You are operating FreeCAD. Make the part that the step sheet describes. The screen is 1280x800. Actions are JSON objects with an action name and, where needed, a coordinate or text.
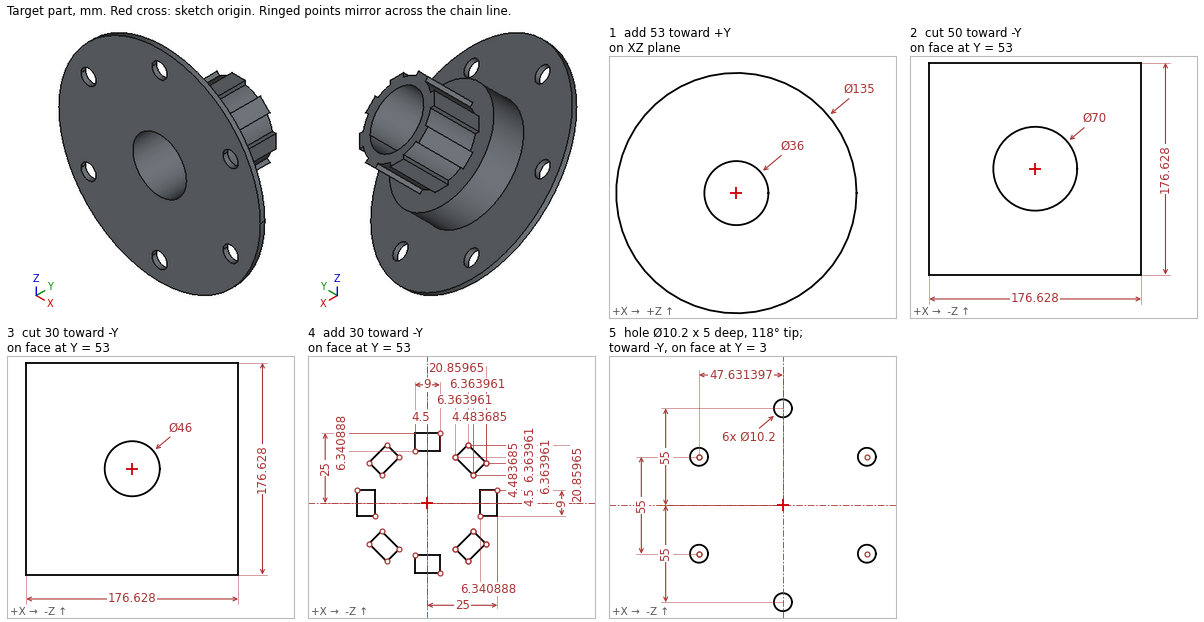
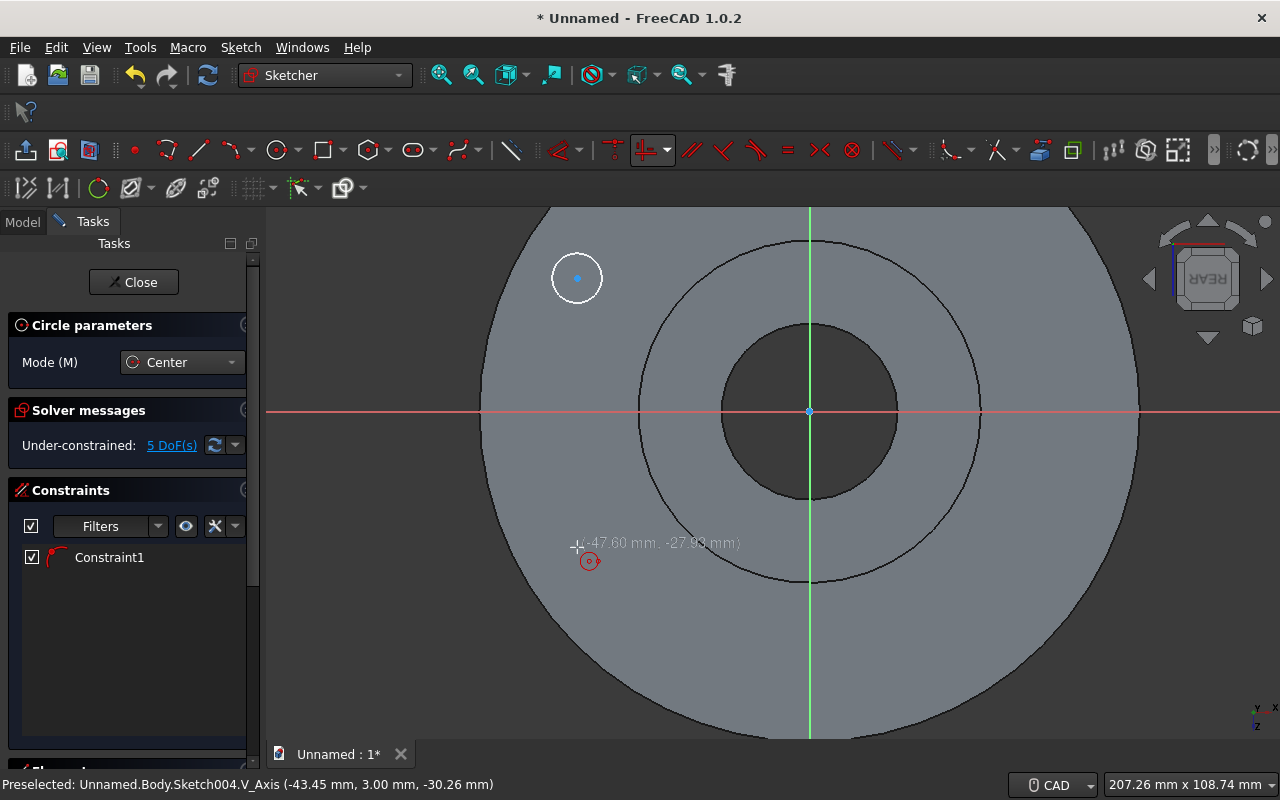
{"action": "left_click", "coordinate": [577, 546]}
{"action": "left_click", "coordinate": [594, 529]}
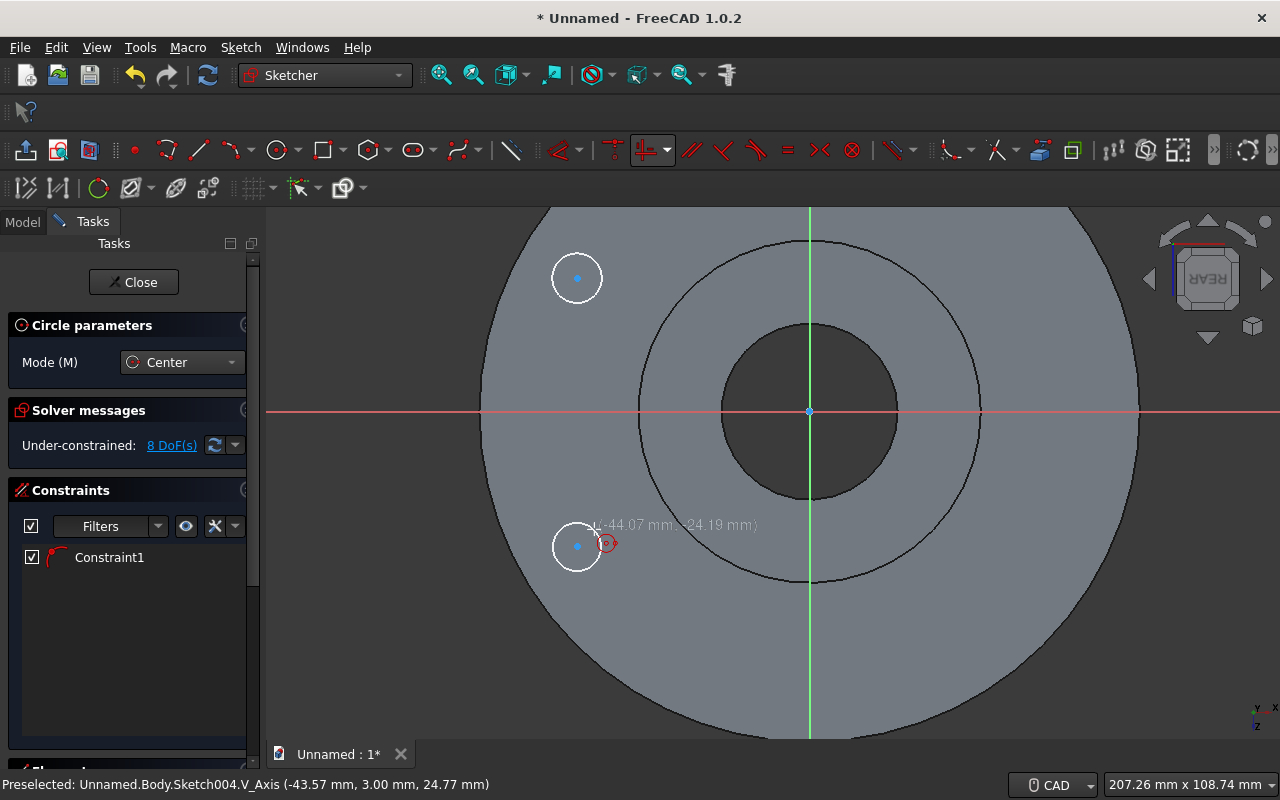
{"action": "left_click", "coordinate": [810, 681]}
{"action": "left_click", "coordinate": [827, 663]}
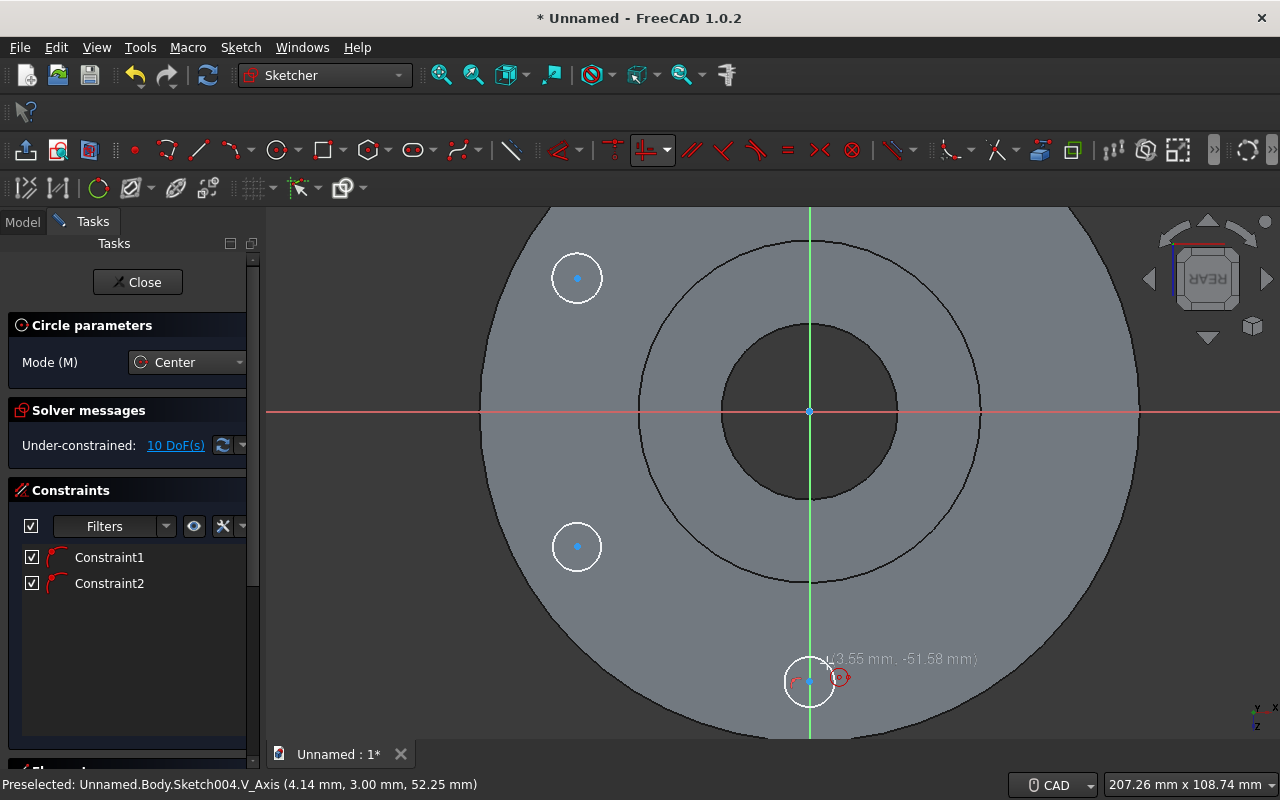
{"action": "left_click", "coordinate": [1043, 546]}
{"action": "left_click", "coordinate": [1060, 529]}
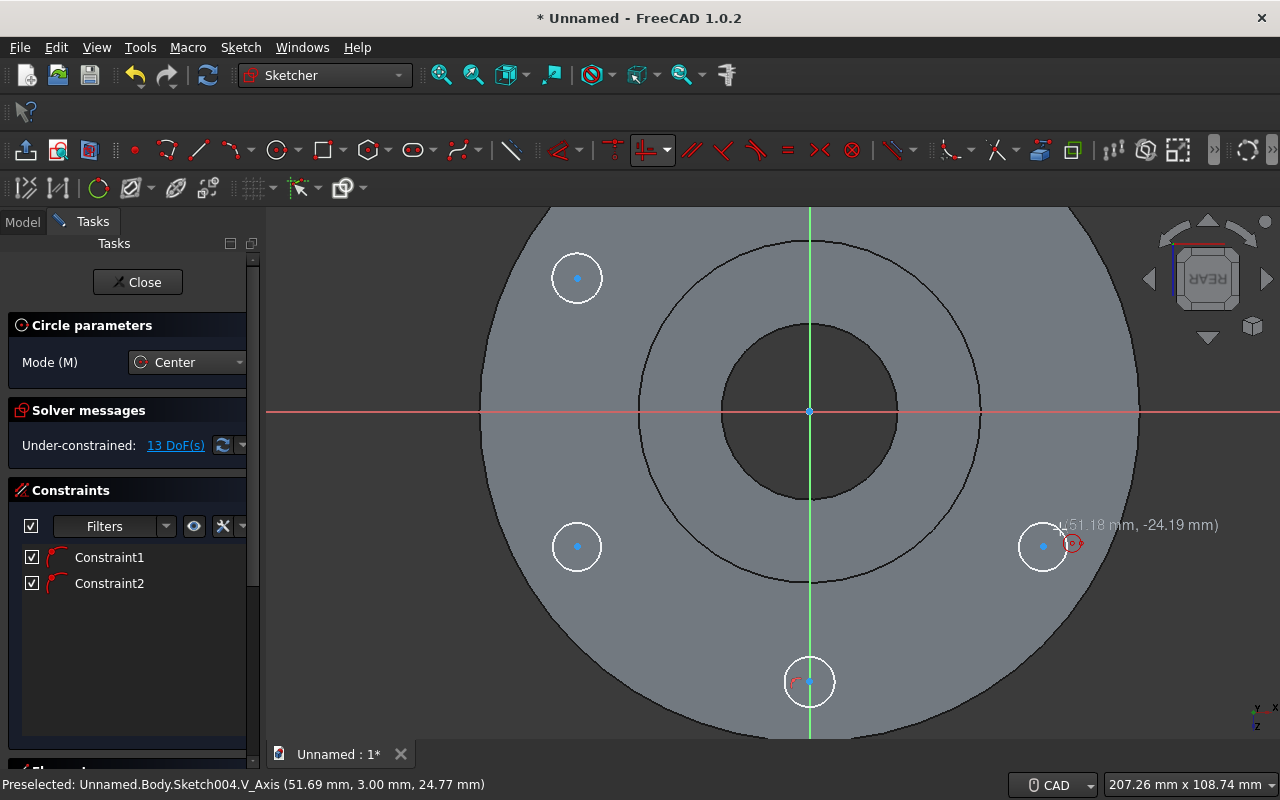
{"action": "left_click", "coordinate": [1043, 277]}
{"action": "left_click", "coordinate": [1060, 259]}
{"action": "key", "text": "Escape"}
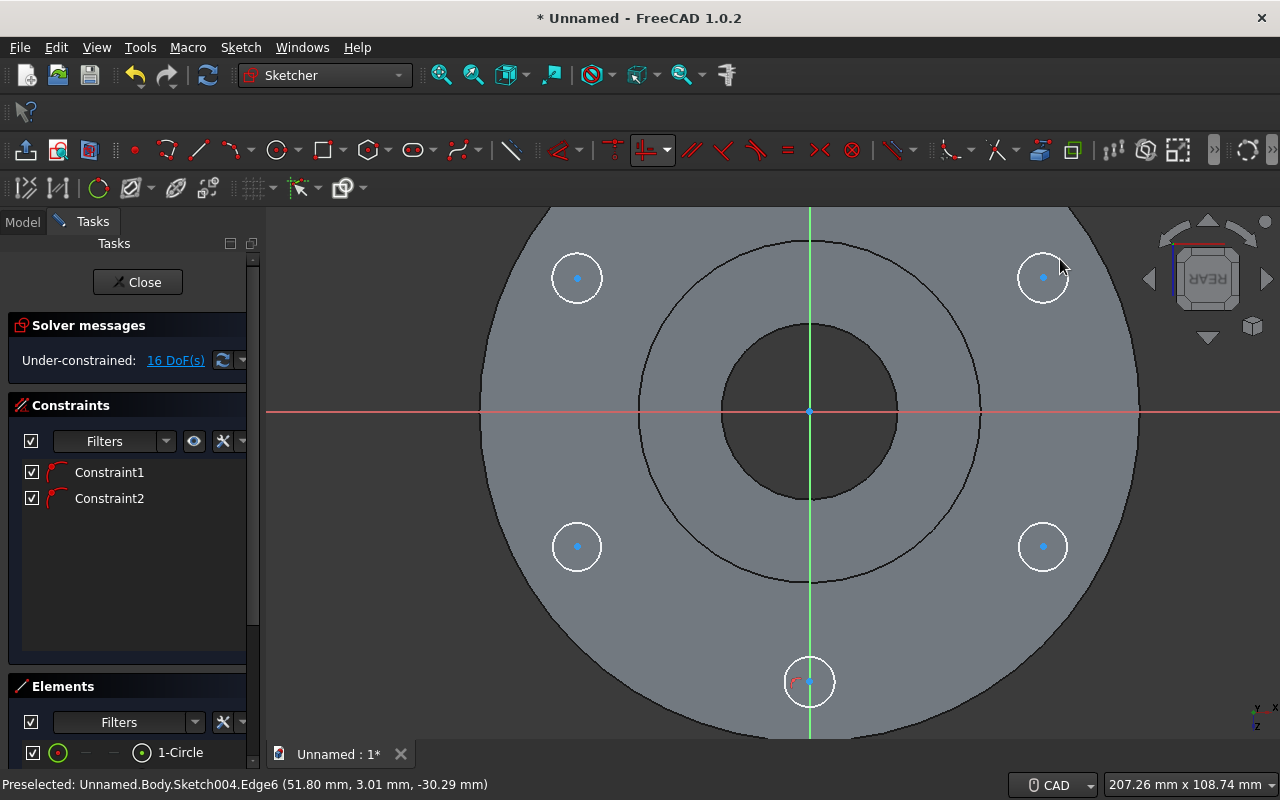
{"action": "scroll", "coordinate": [577, 548], "scroll_direction": "down", "scroll_amount": 3}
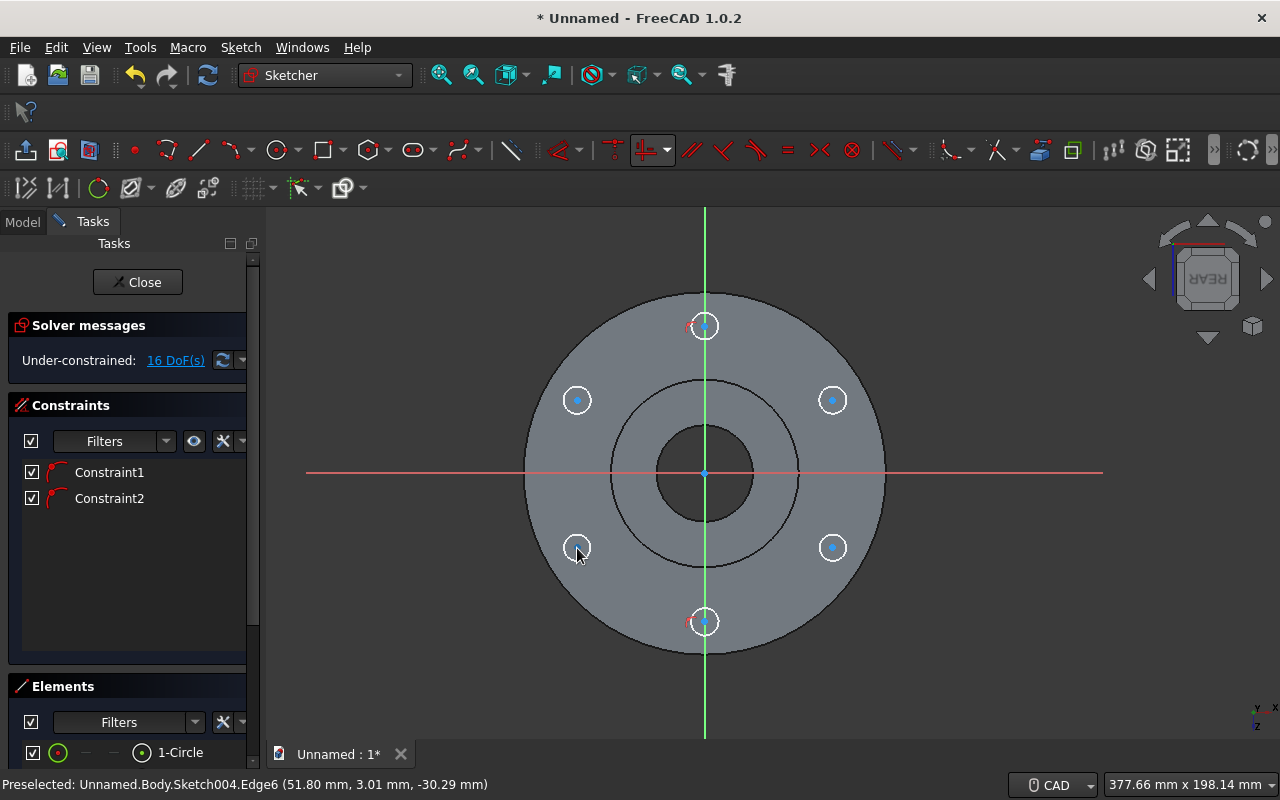
{"action": "scroll", "coordinate": [714, 317], "scroll_direction": "up", "scroll_amount": 2}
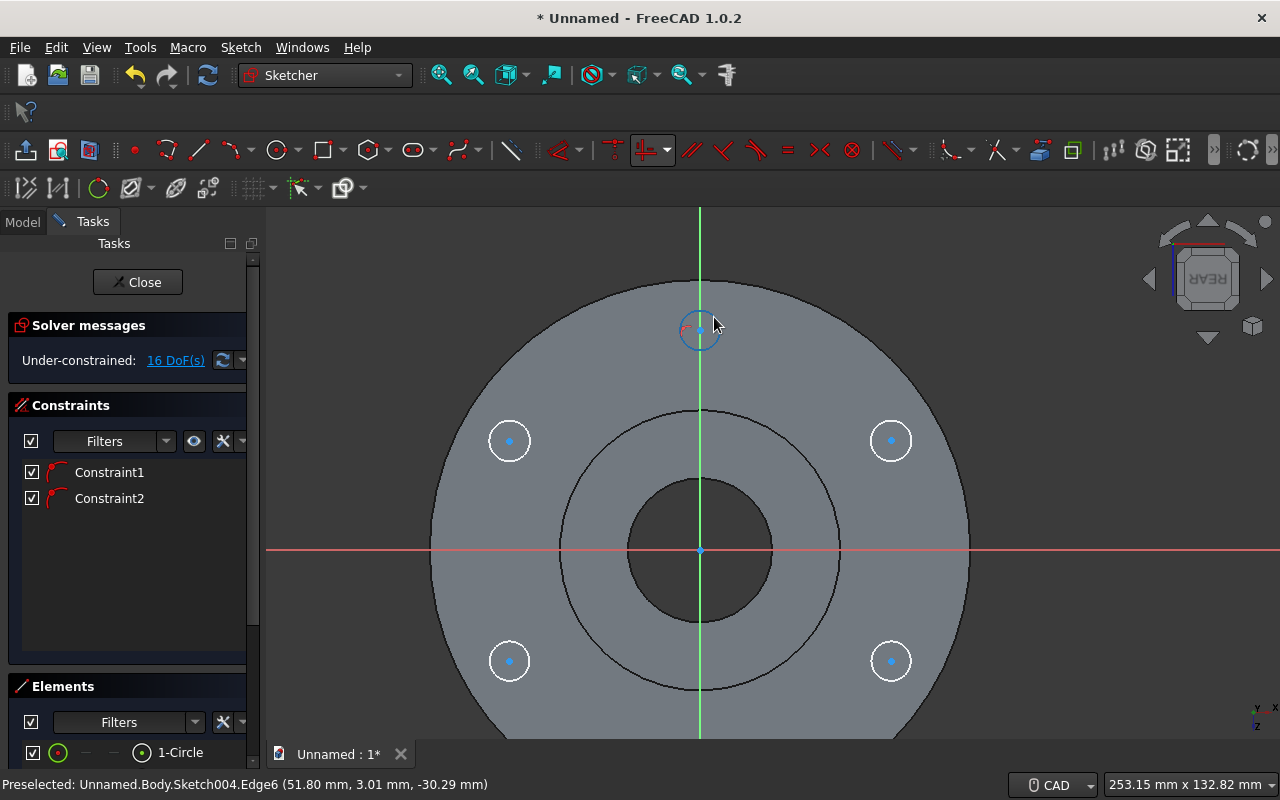
{"action": "left_click", "coordinate": [714, 316]}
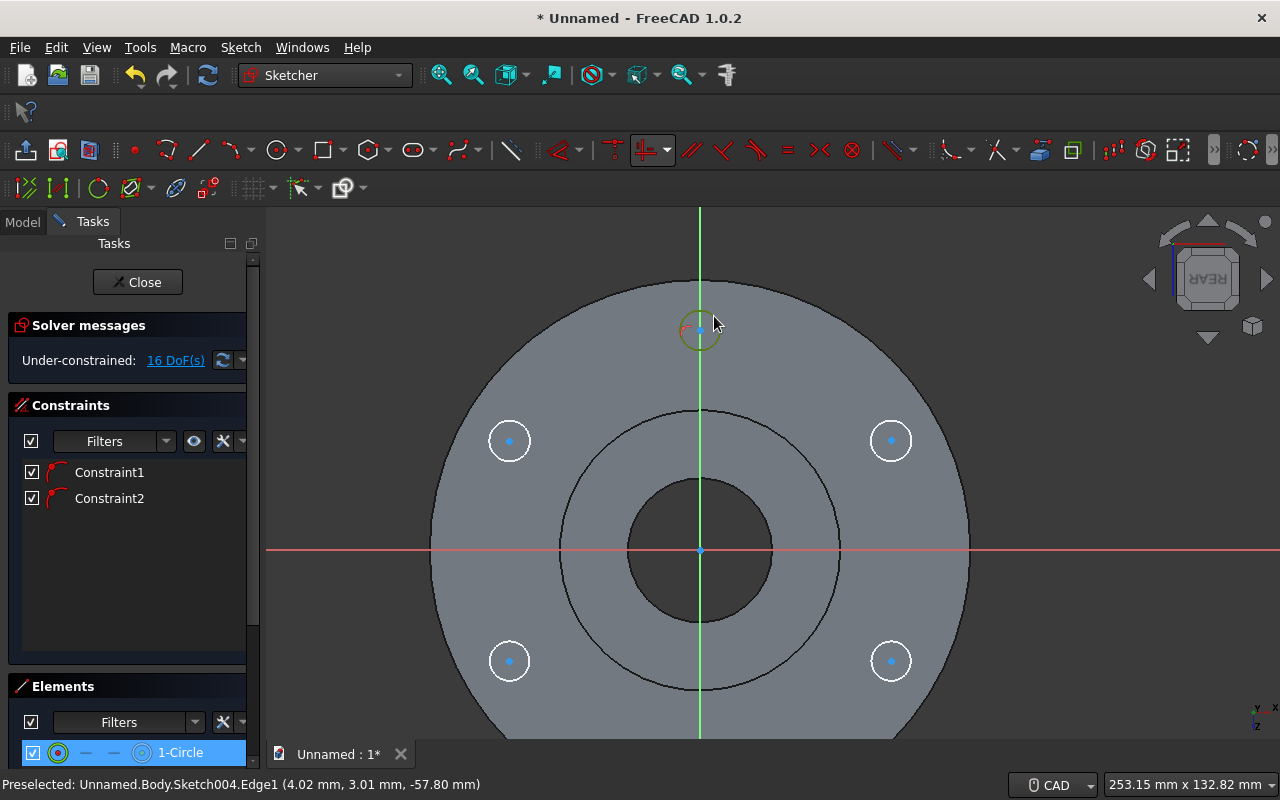
{"action": "left_click", "coordinate": [524, 427]}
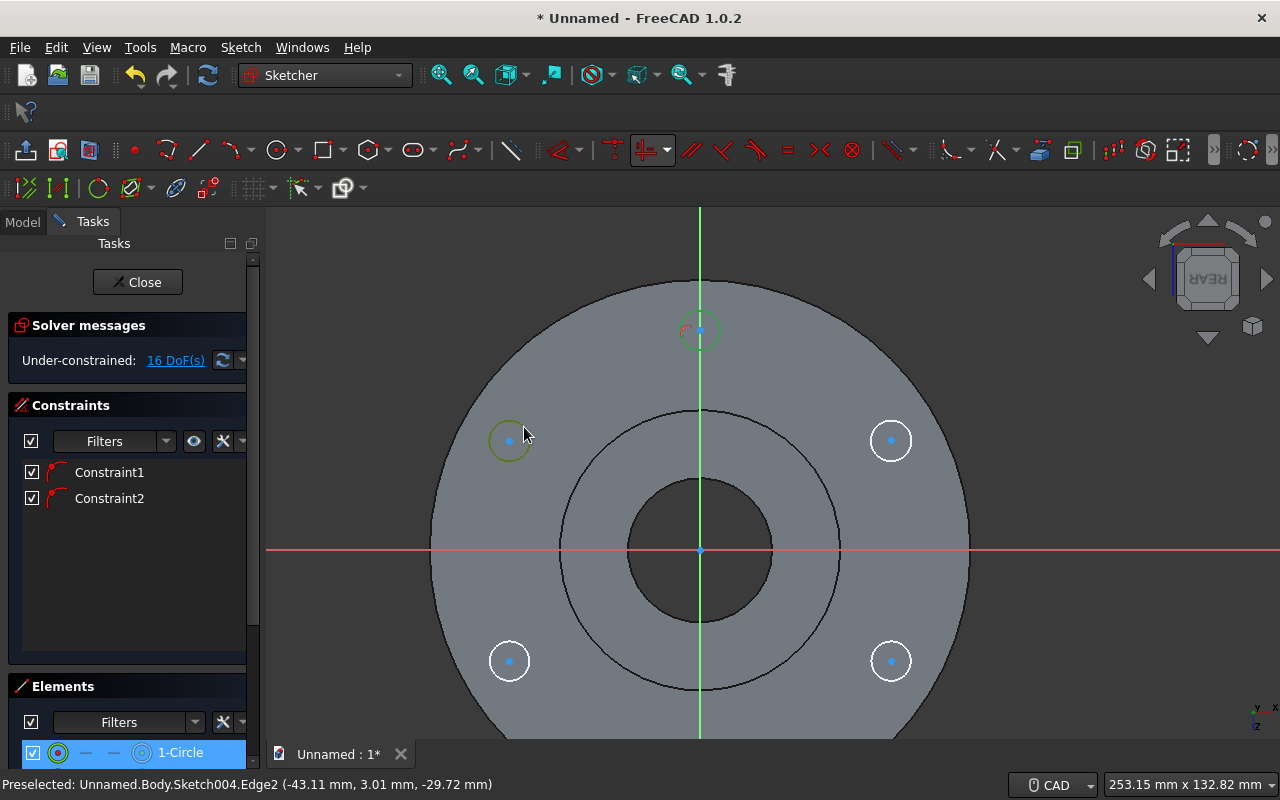
{"action": "left_click", "coordinate": [523, 647]}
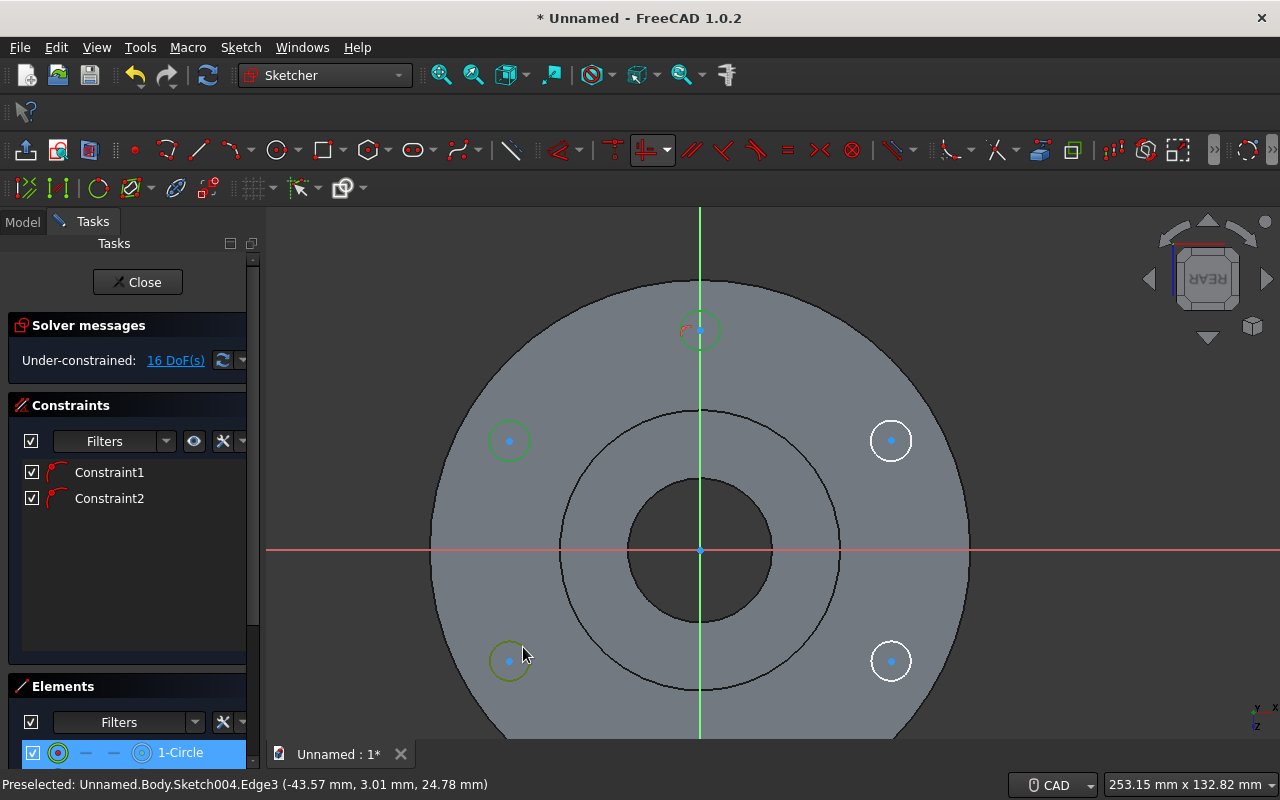
{"action": "scroll", "coordinate": [714, 316], "scroll_direction": "down", "scroll_amount": 2}